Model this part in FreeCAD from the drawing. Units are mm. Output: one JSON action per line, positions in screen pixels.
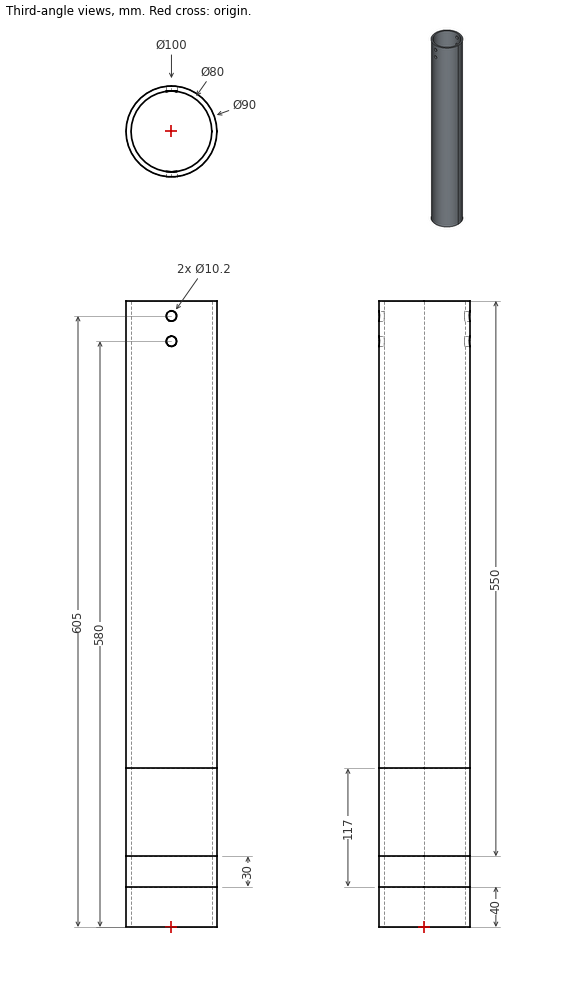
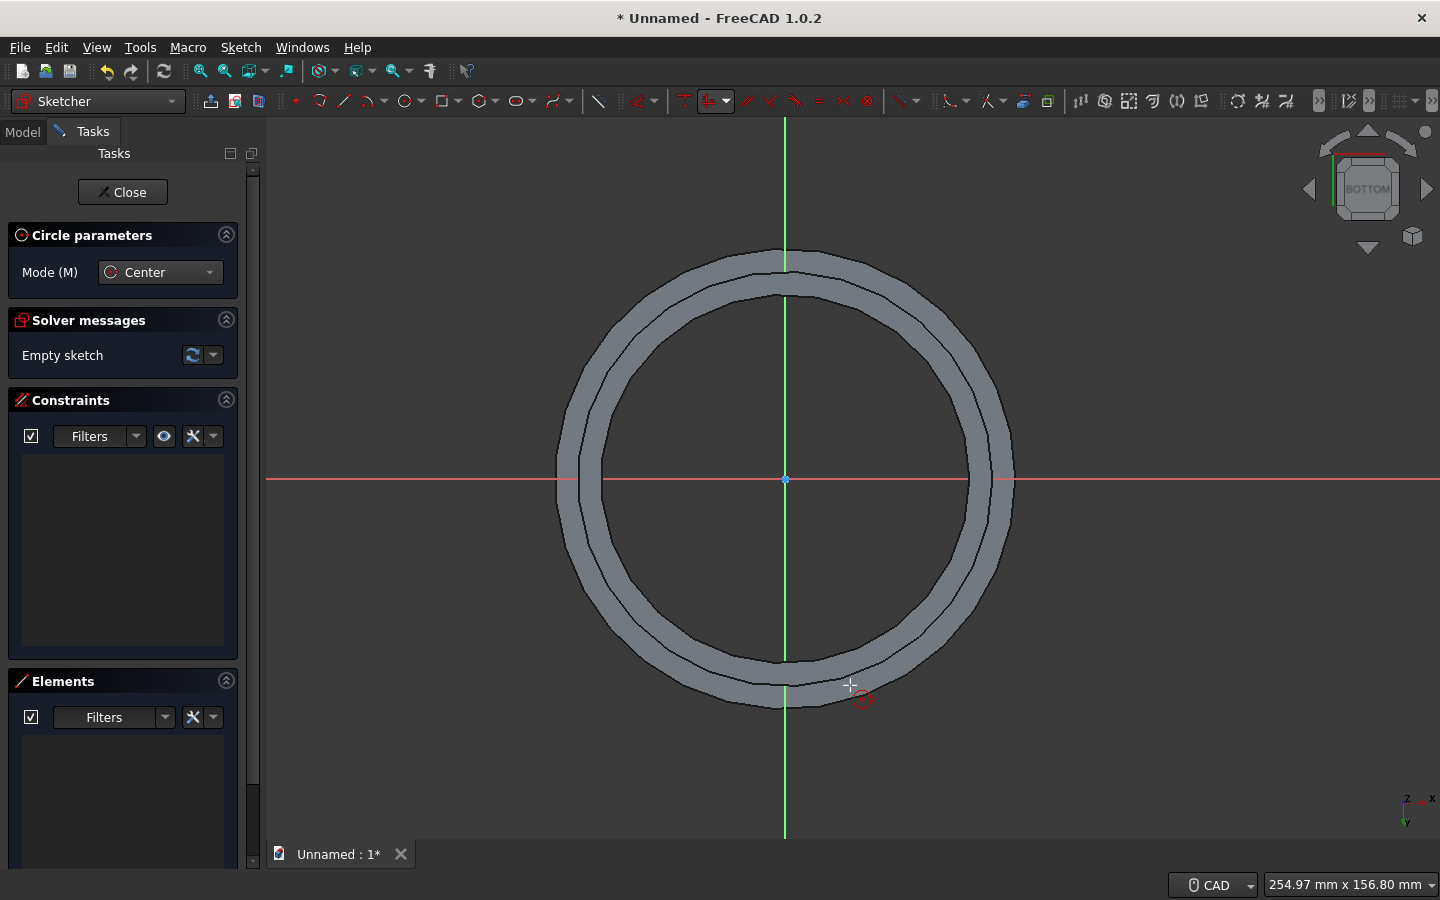
{"action": "left_click", "coordinate": [785, 479]}
{"action": "mouse_move", "coordinate": [948, 316]}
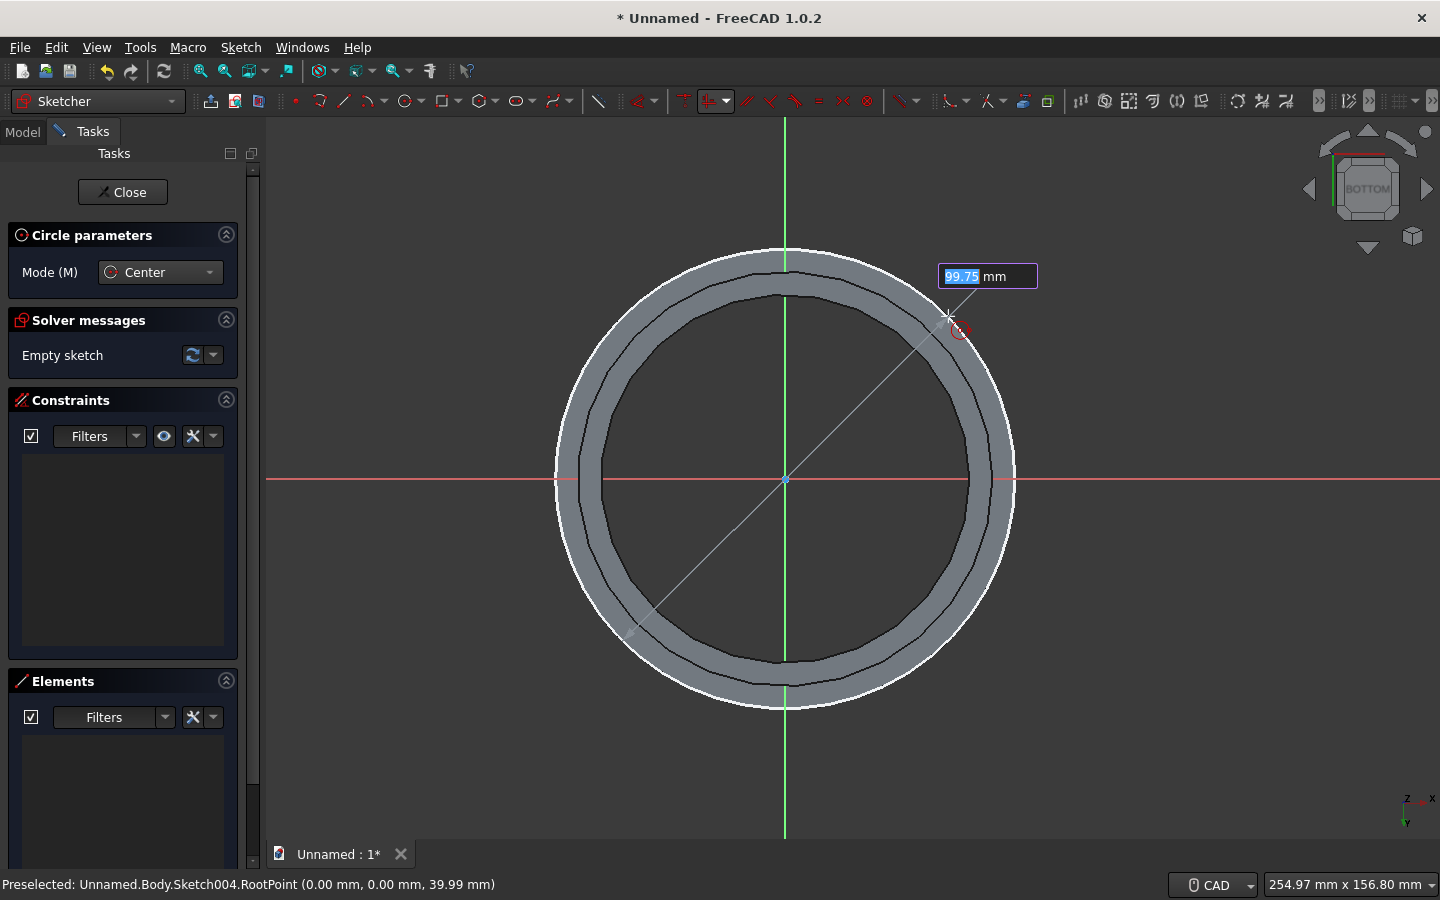
{"action": "type", "text": "100"}
{"action": "key", "text": "Return"}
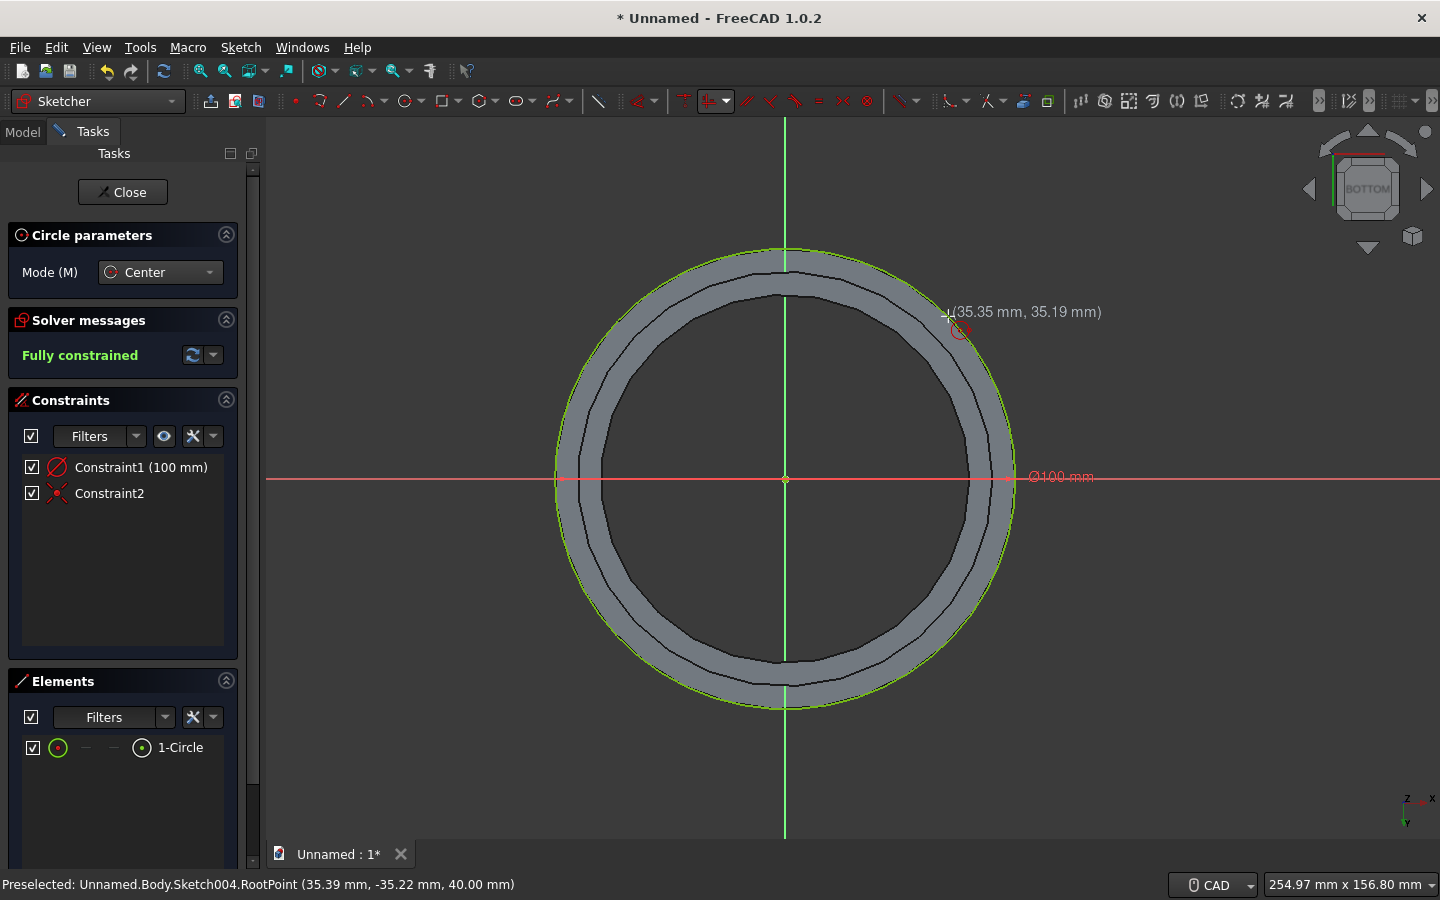
{"action": "left_click", "coordinate": [785, 479]}
{"action": "mouse_move", "coordinate": [932, 332]}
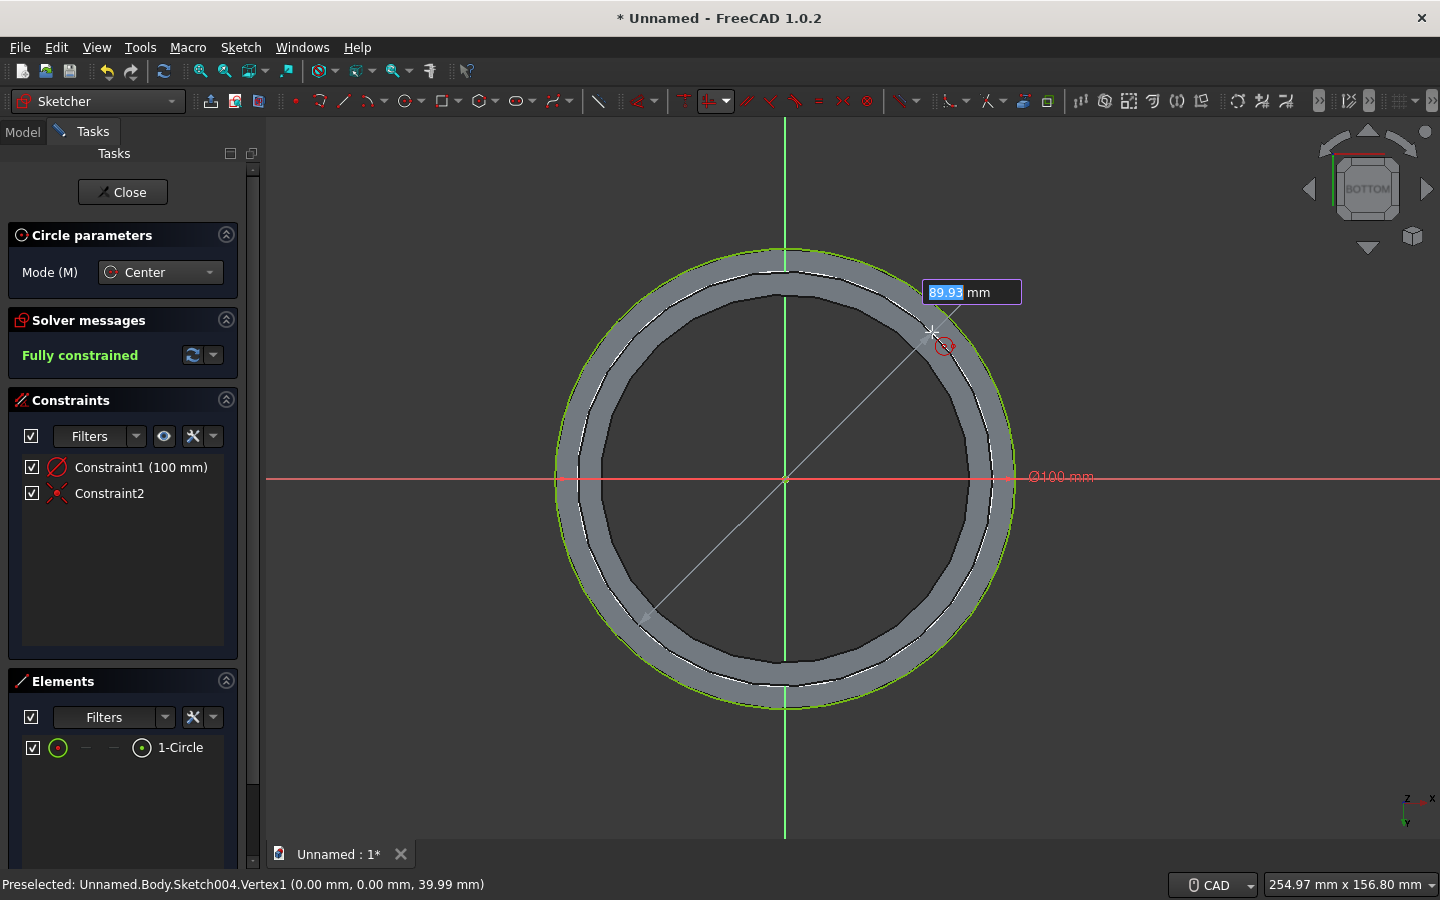
{"action": "type", "text": "90"}
{"action": "key", "text": "Return"}
{"action": "key", "text": "Escape"}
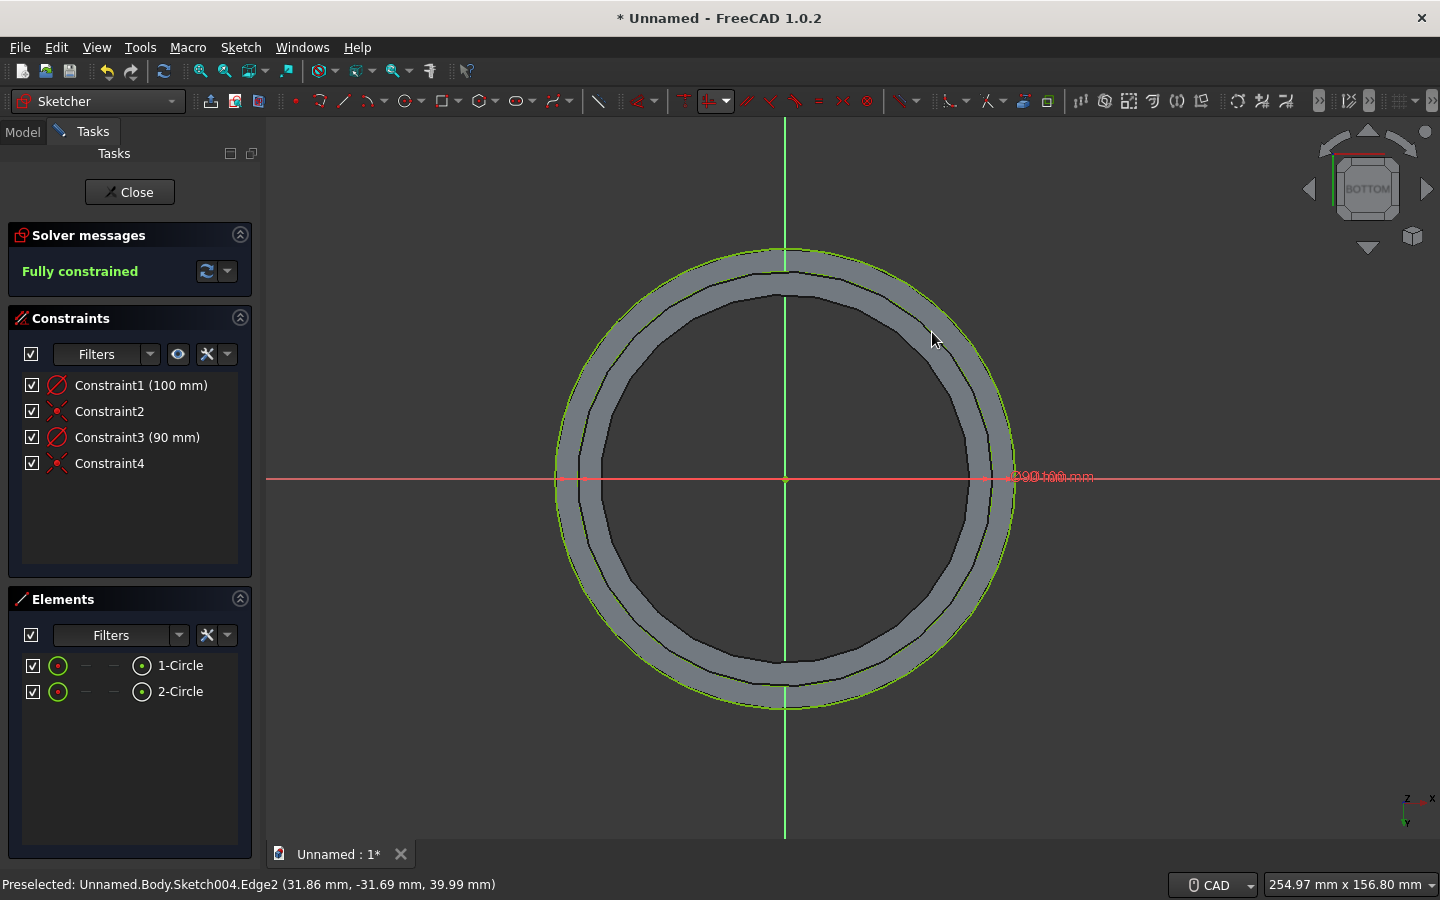
{"action": "left_click", "coordinate": [130, 192]}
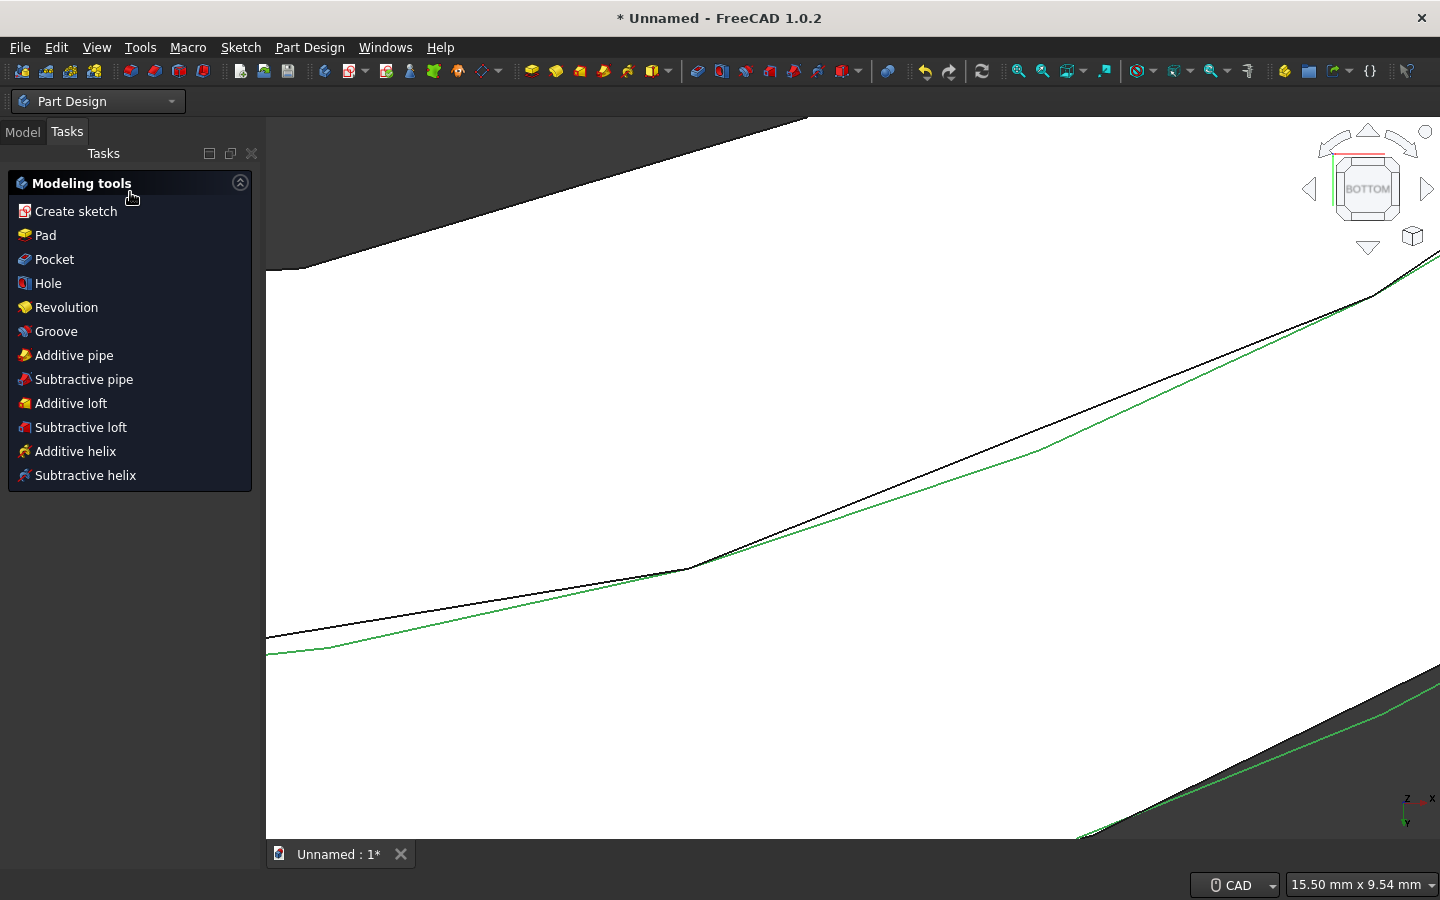
{"action": "left_click", "coordinate": [698, 72]}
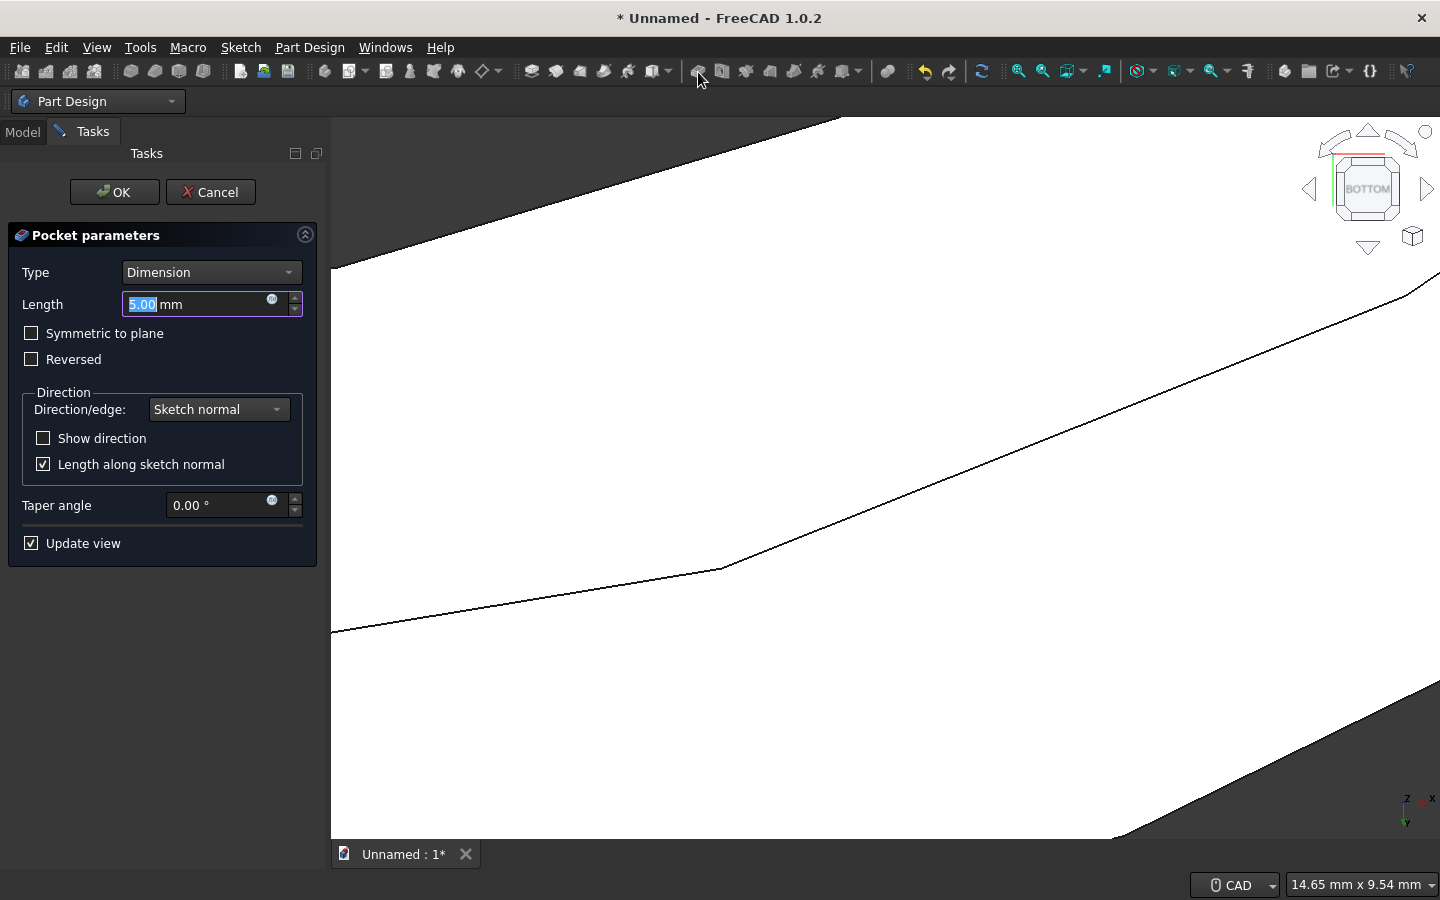
{"action": "type", "text": "117"}
{"action": "key", "text": "Tab"}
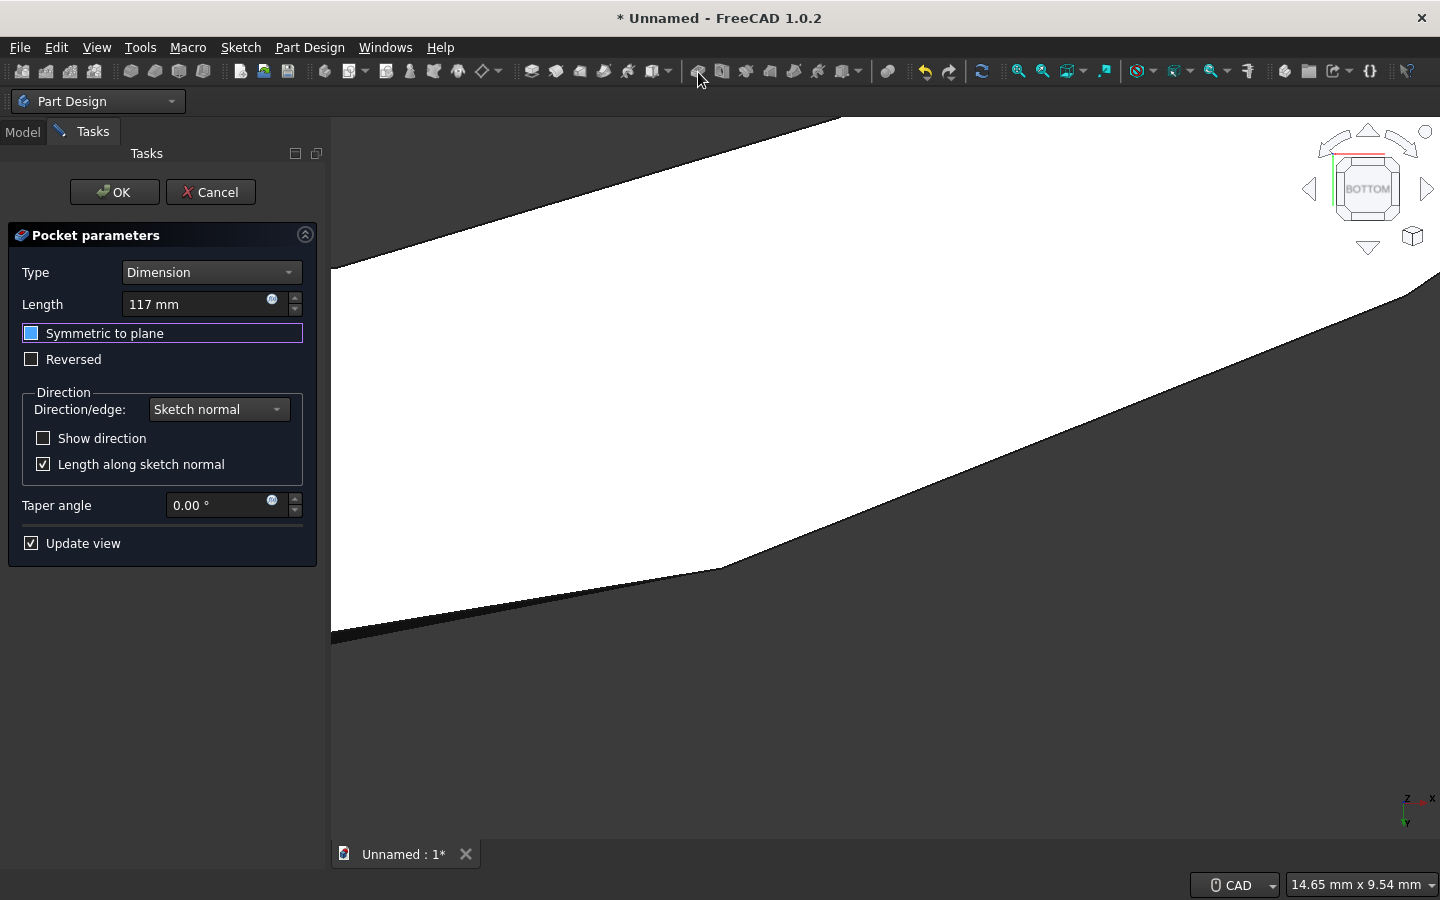
{"action": "left_click", "coordinate": [115, 192]}